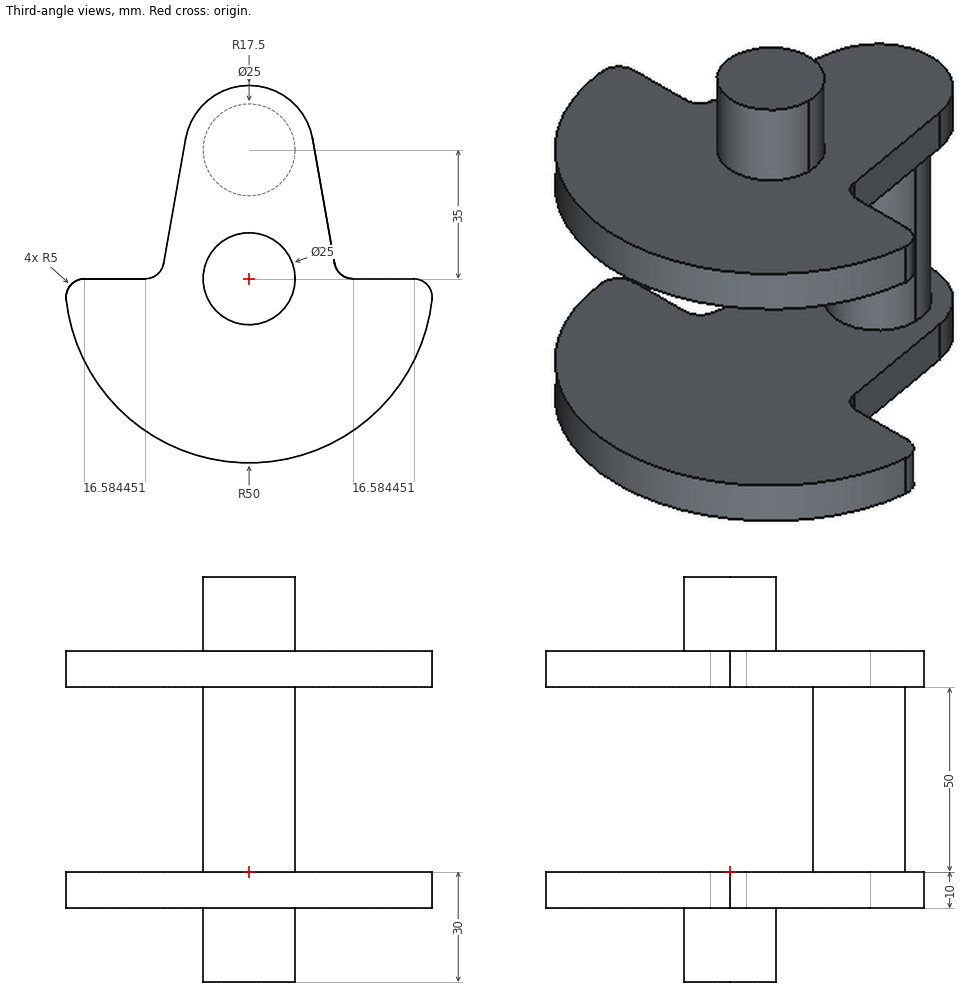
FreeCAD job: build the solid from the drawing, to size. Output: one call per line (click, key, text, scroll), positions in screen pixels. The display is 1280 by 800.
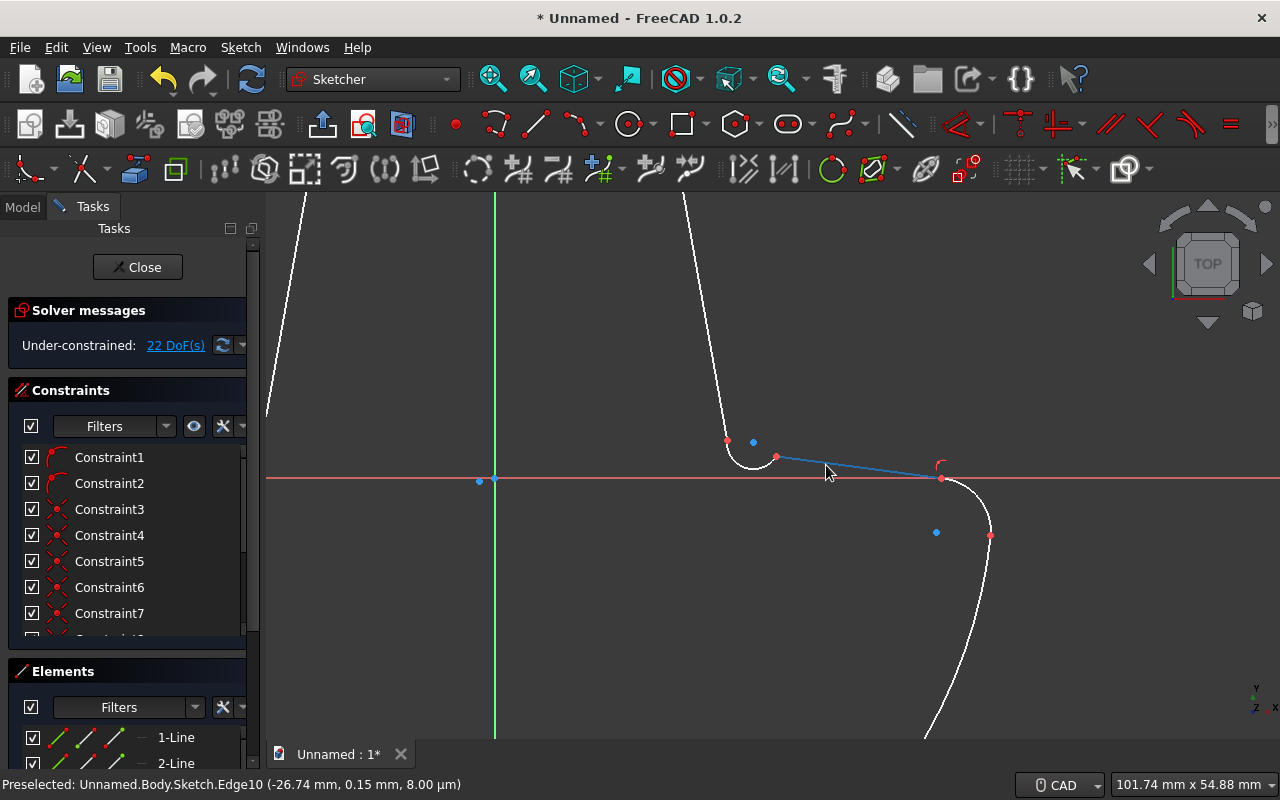
click(826, 463)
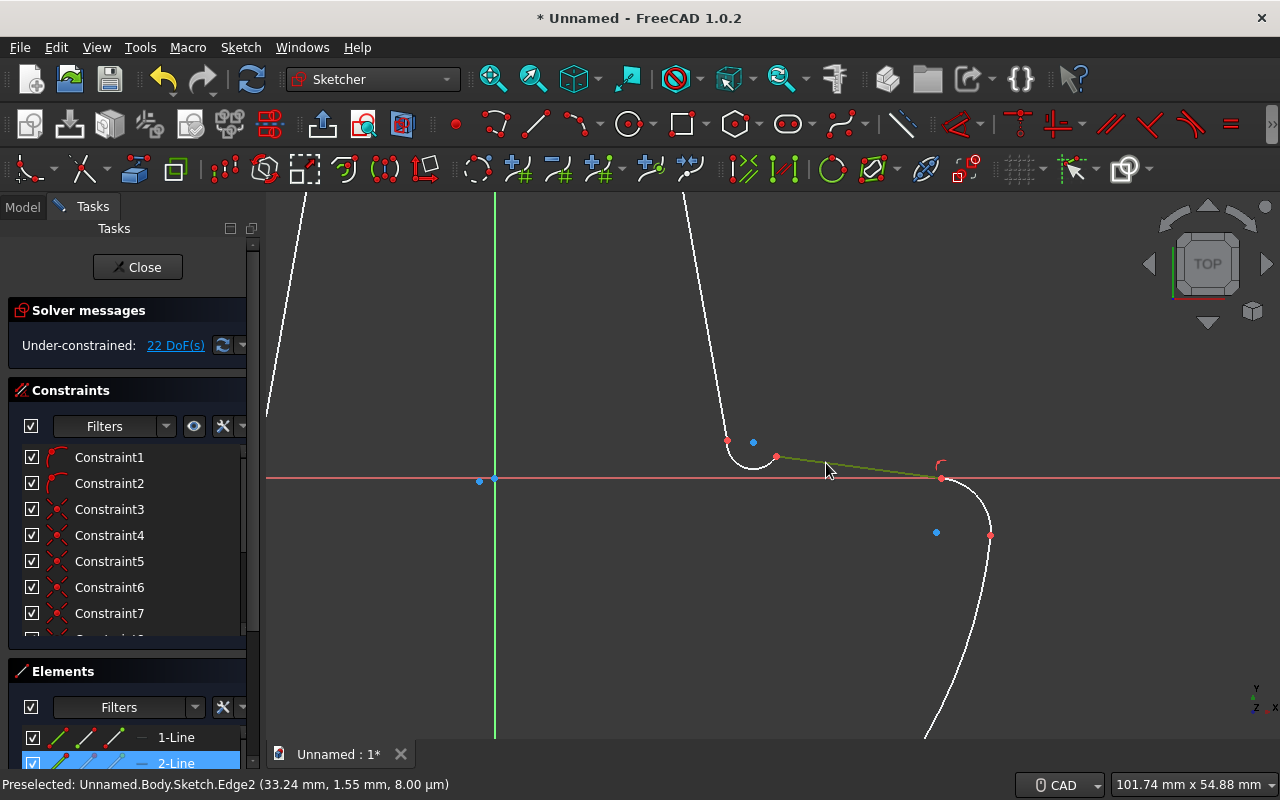
click(987, 511)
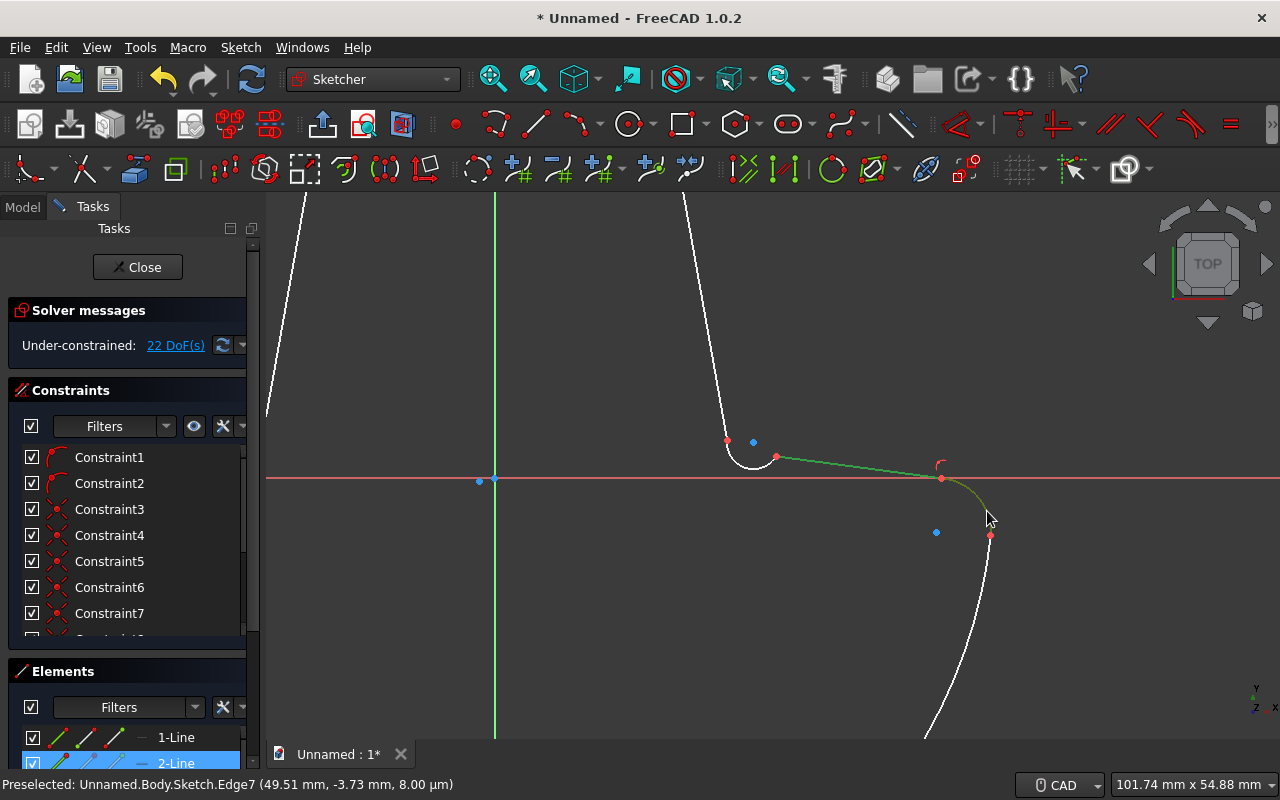
click(1192, 124)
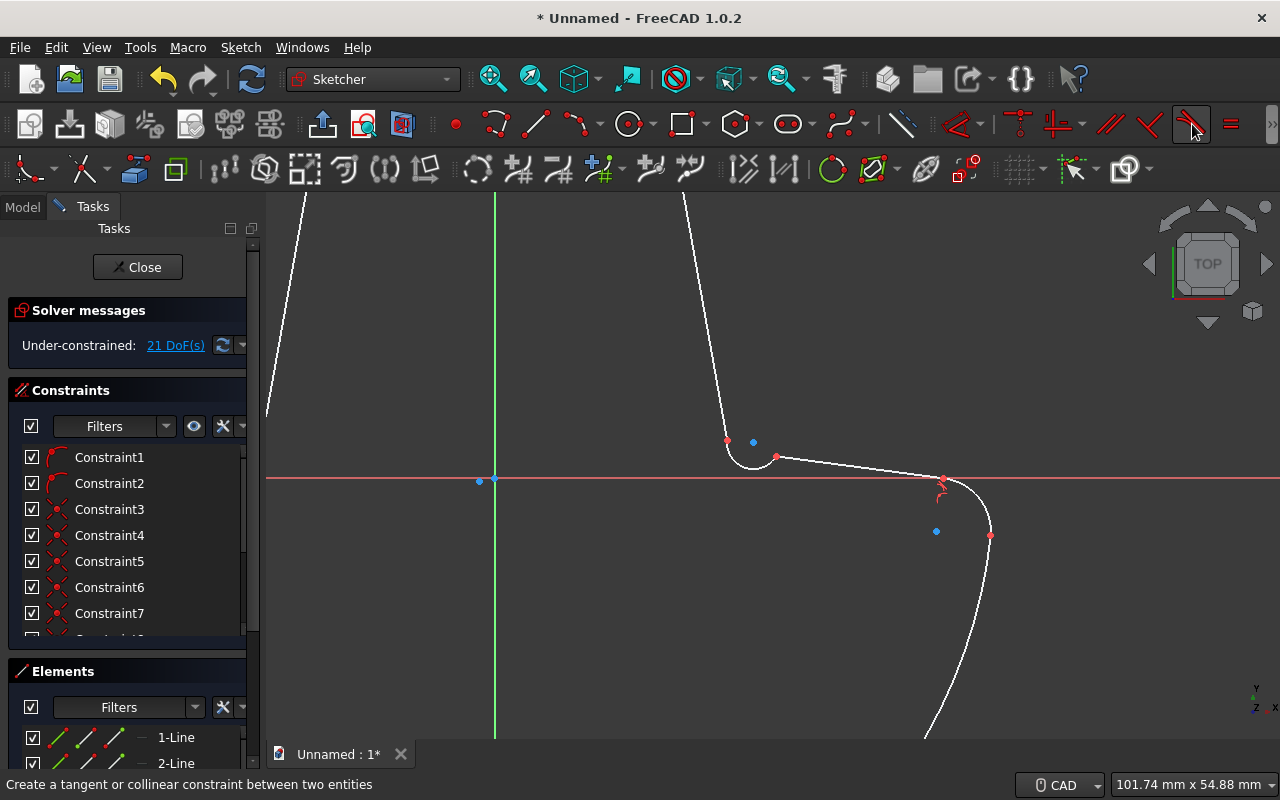
click(826, 463)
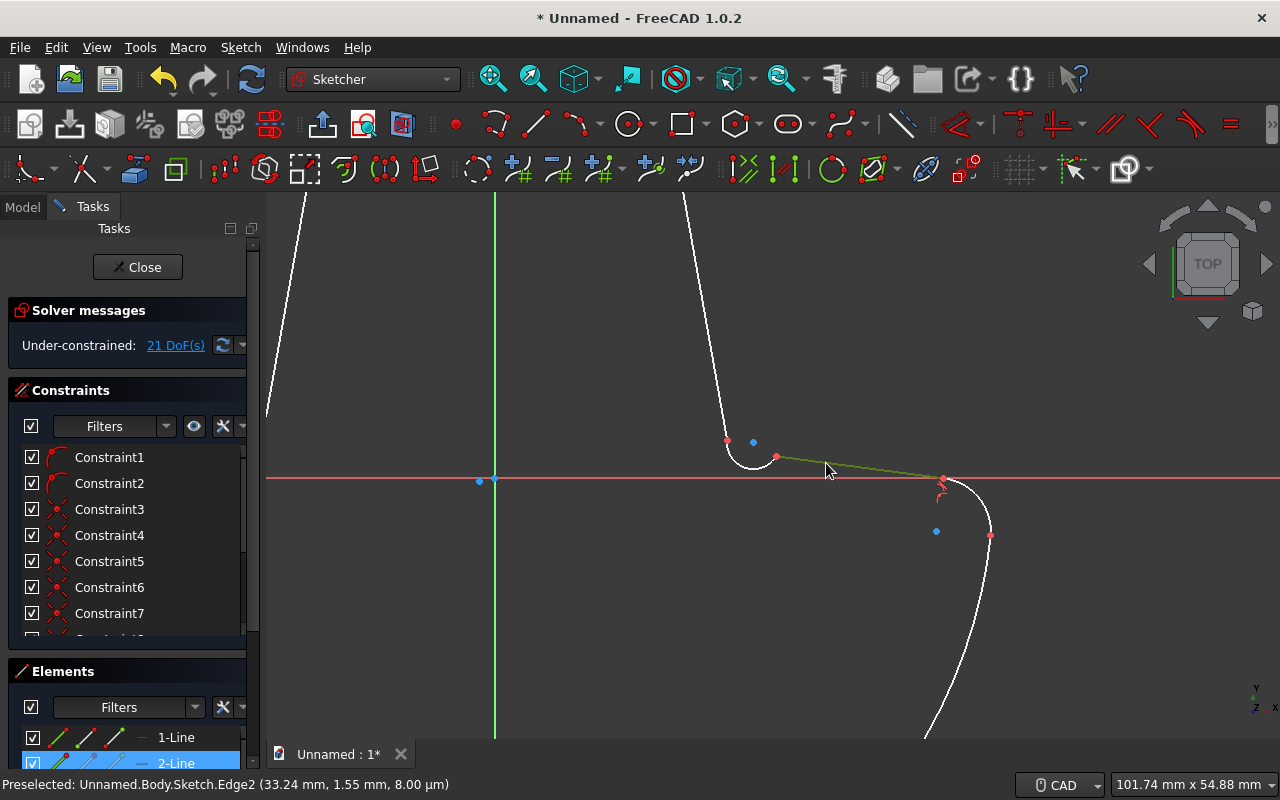
click(733, 460)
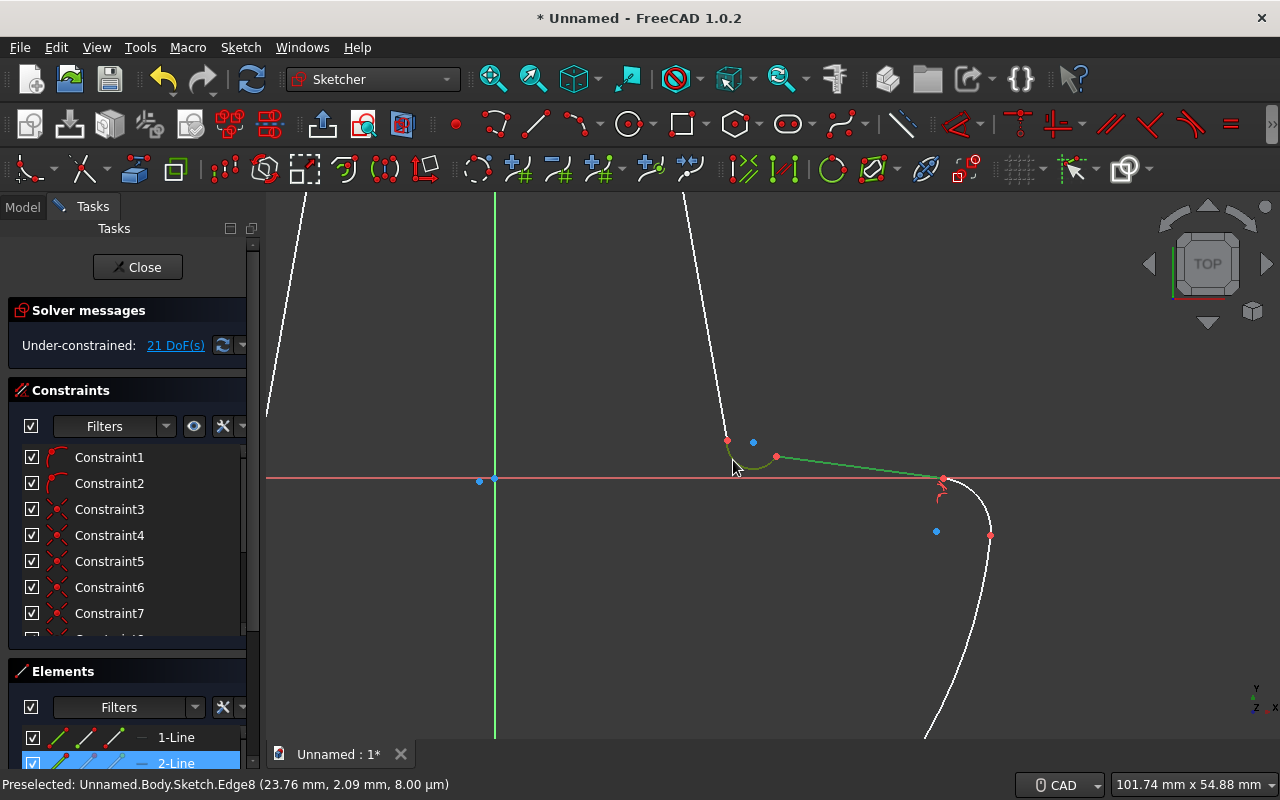
click(1192, 124)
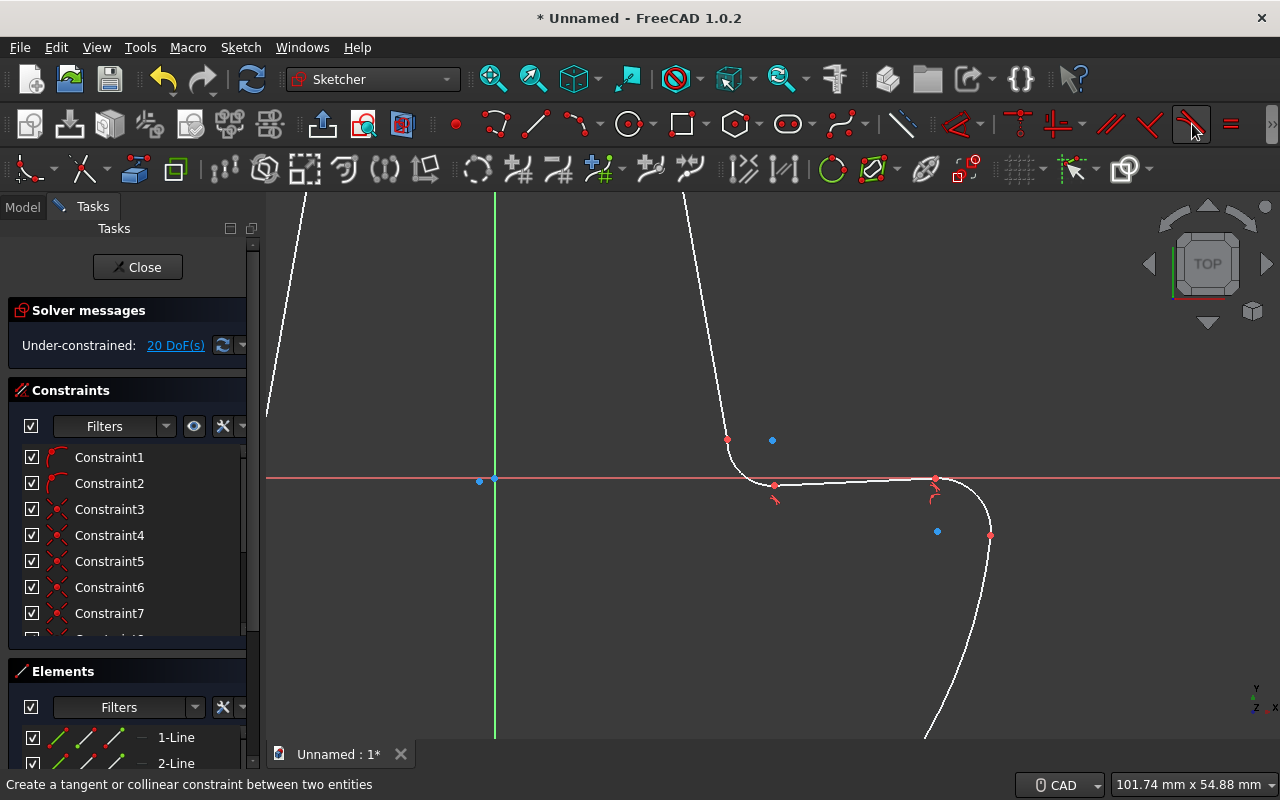
click(709, 339)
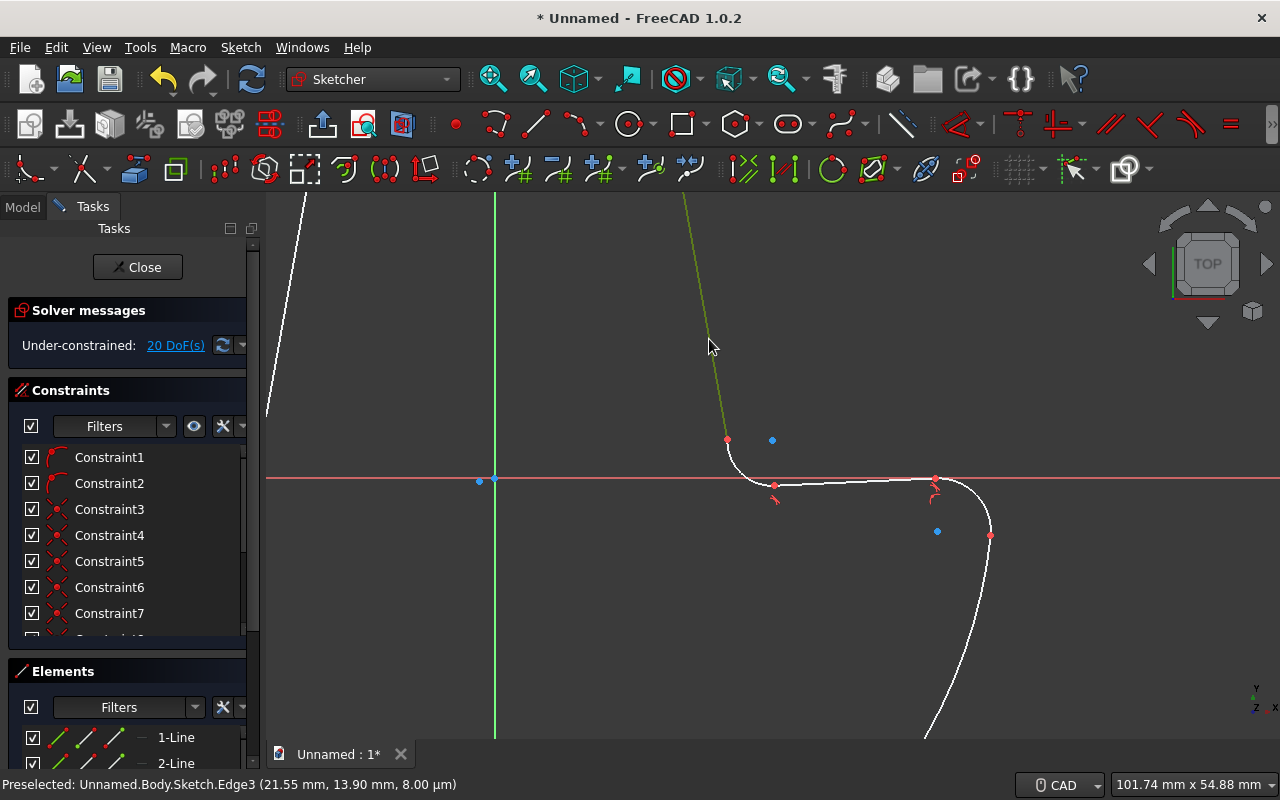
click(732, 461)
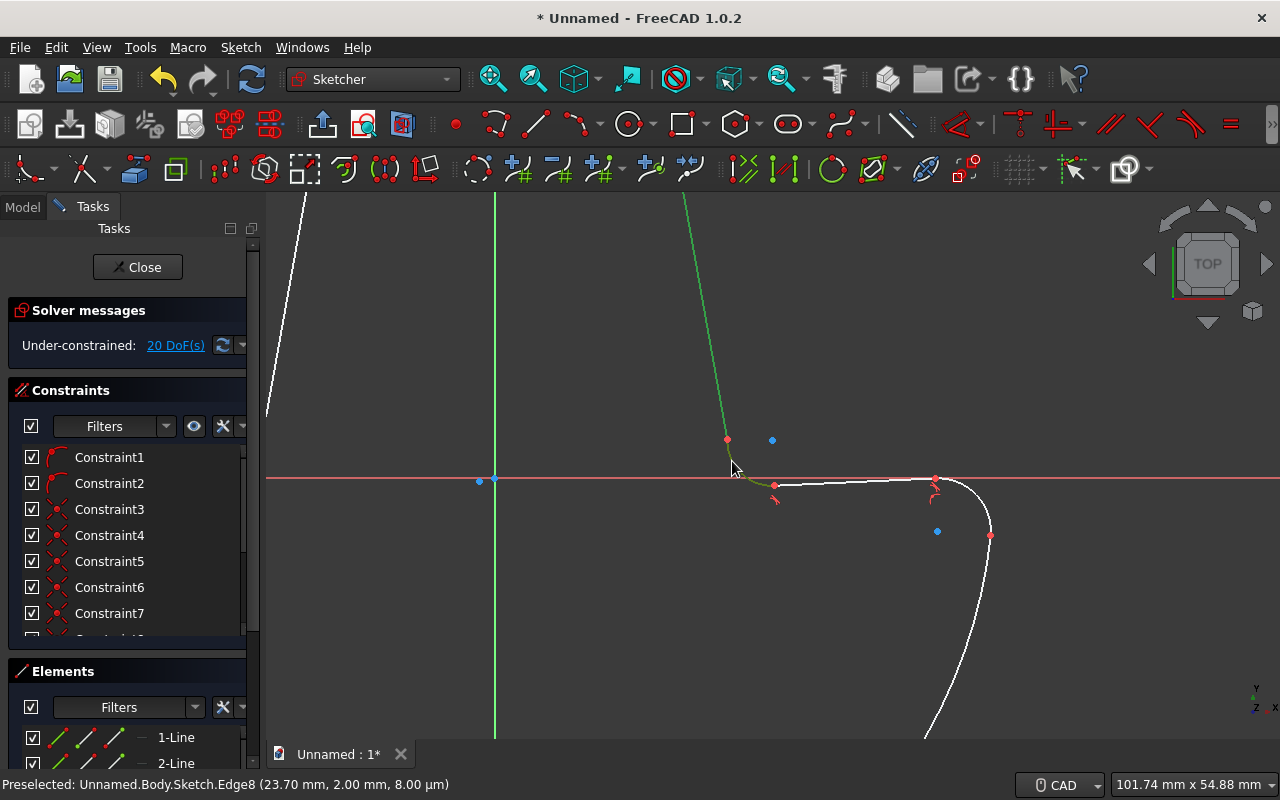
key(t)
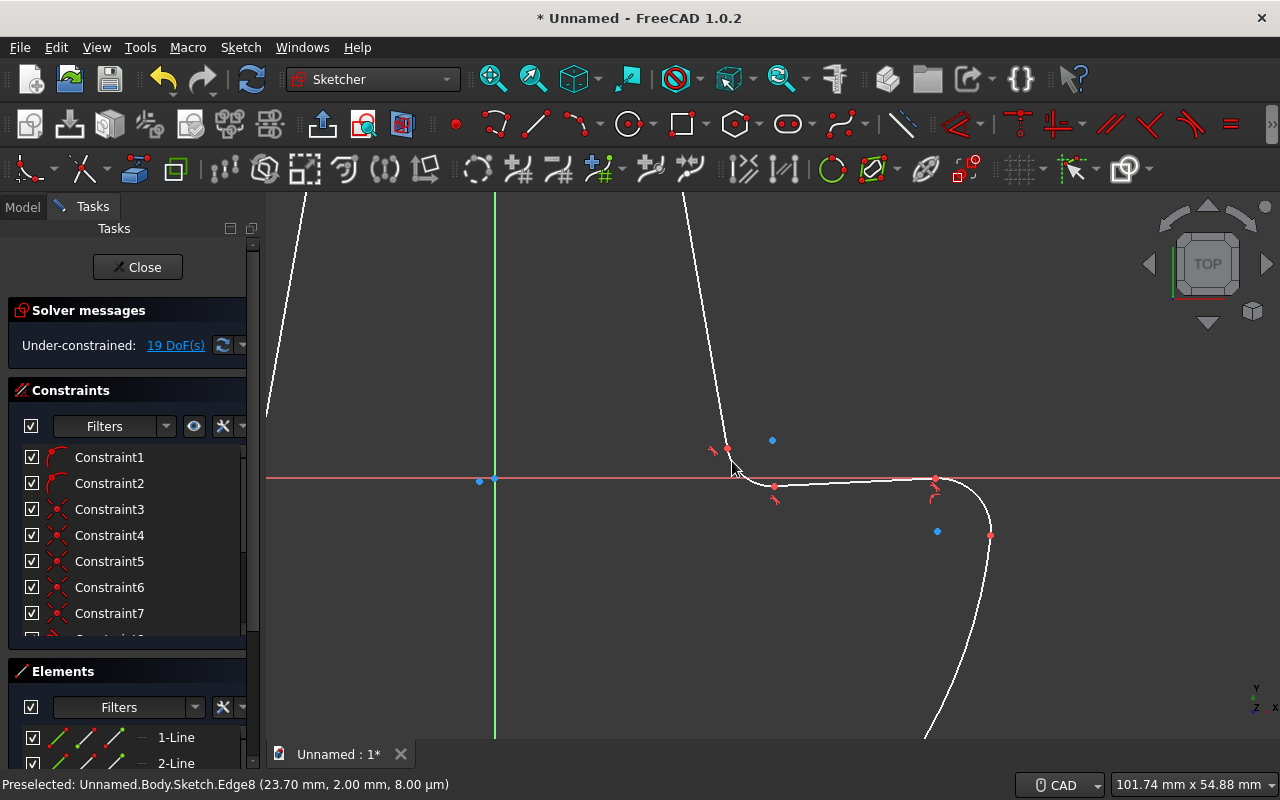
click(709, 345)